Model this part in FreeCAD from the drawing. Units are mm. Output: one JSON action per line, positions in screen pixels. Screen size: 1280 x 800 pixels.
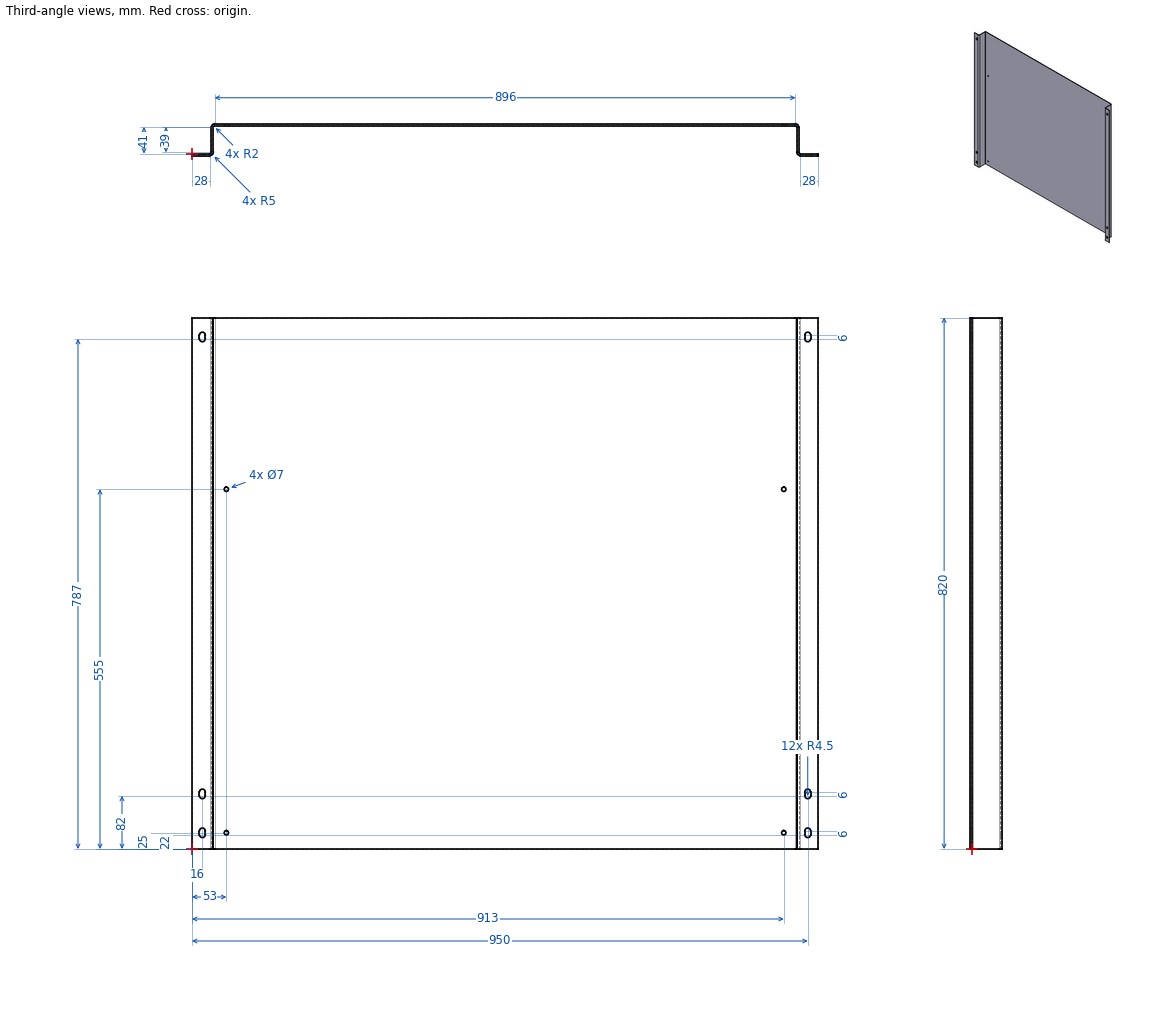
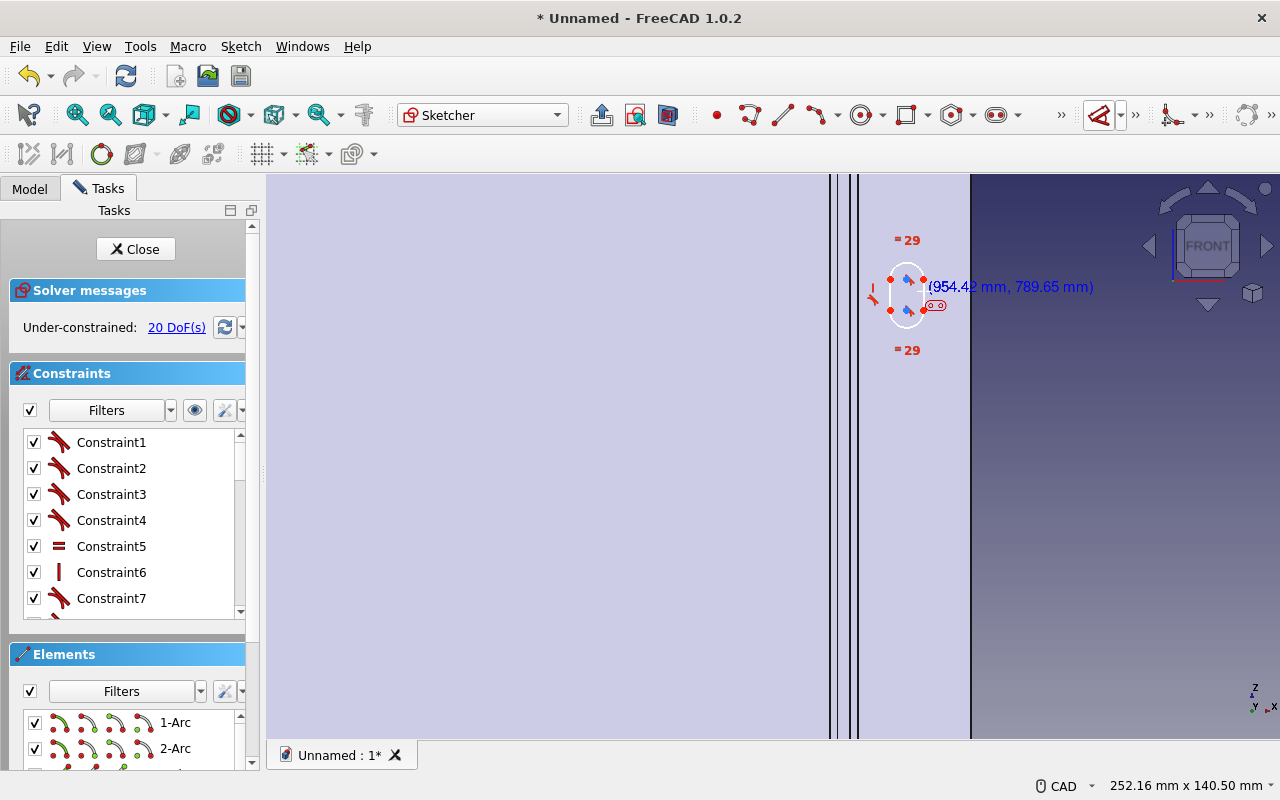
{"action": "scroll", "coordinate": [916, 281], "scroll_direction": "down", "scroll_amount": 11}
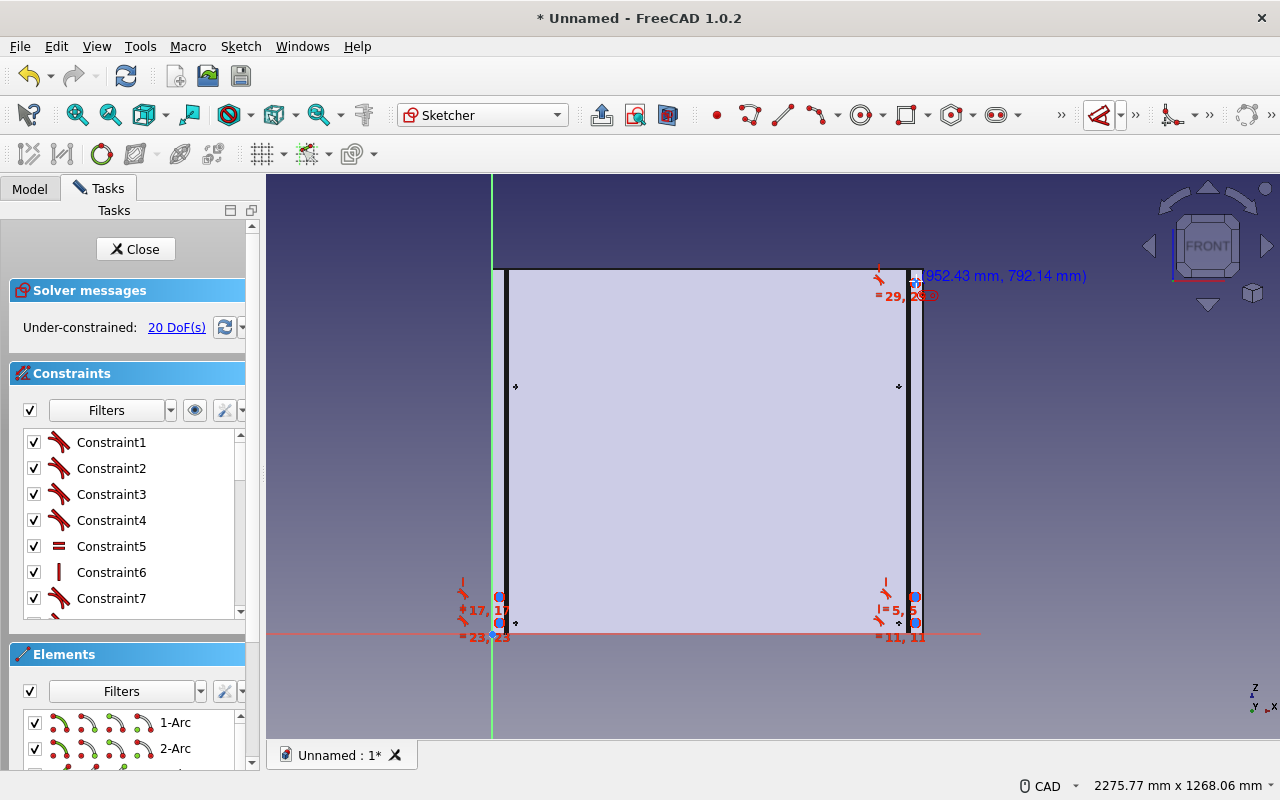
{"action": "scroll", "coordinate": [499, 284], "scroll_direction": "up", "scroll_amount": 13}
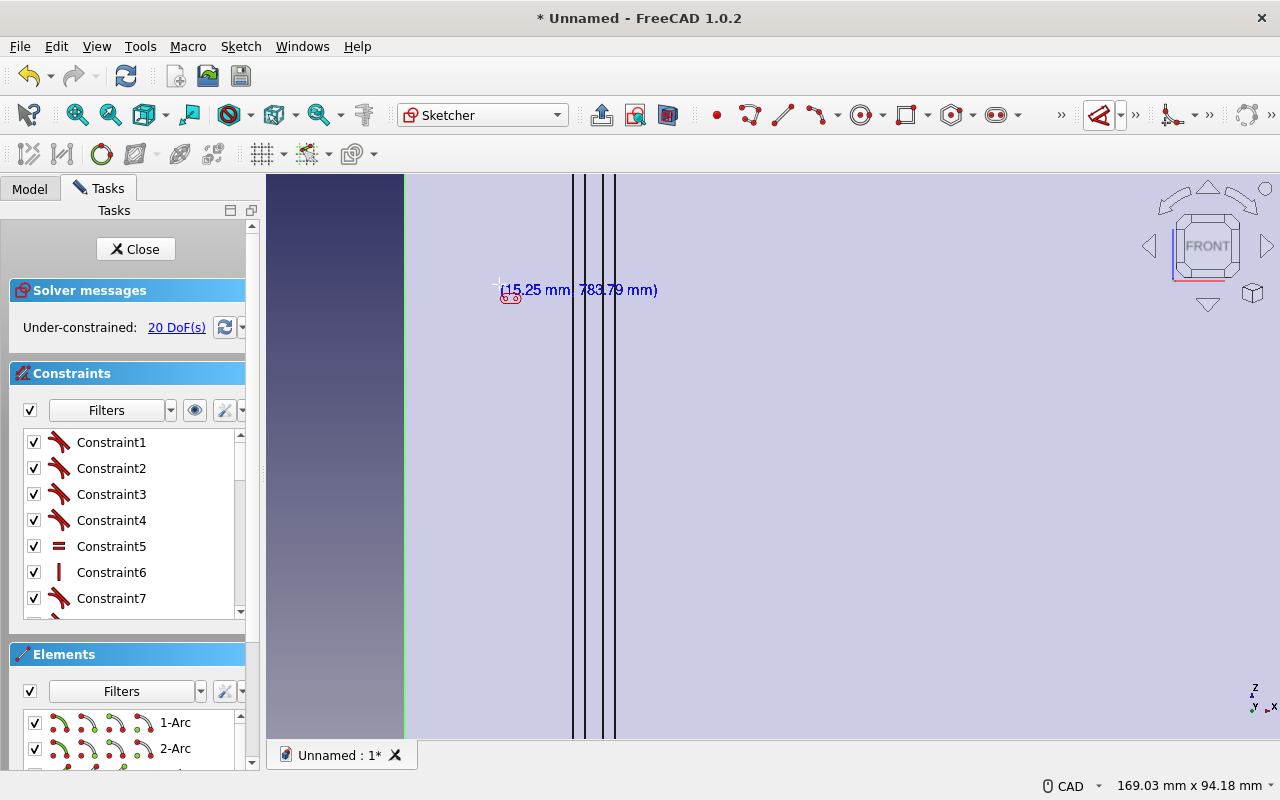
{"action": "scroll", "coordinate": [499, 284], "scroll_direction": "down", "scroll_amount": 13}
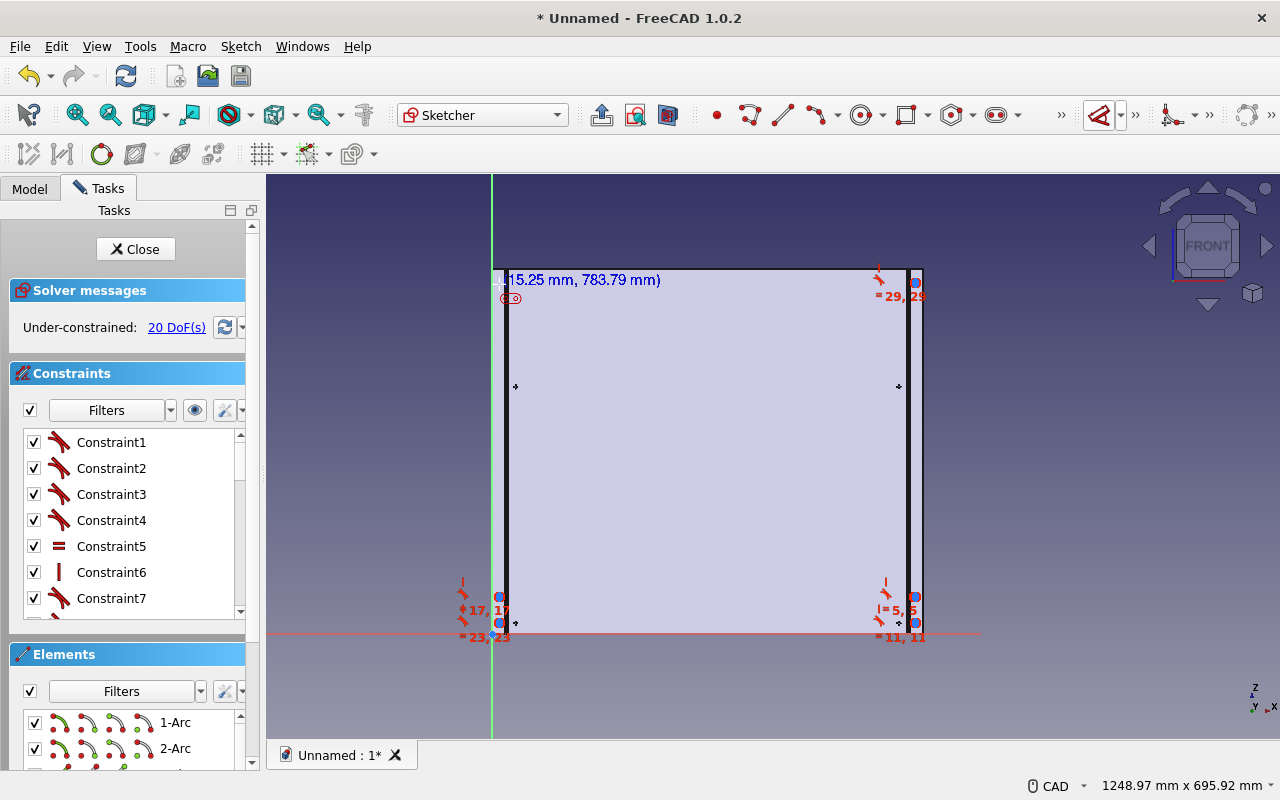
{"action": "scroll", "coordinate": [499, 284], "scroll_direction": "up", "scroll_amount": 5}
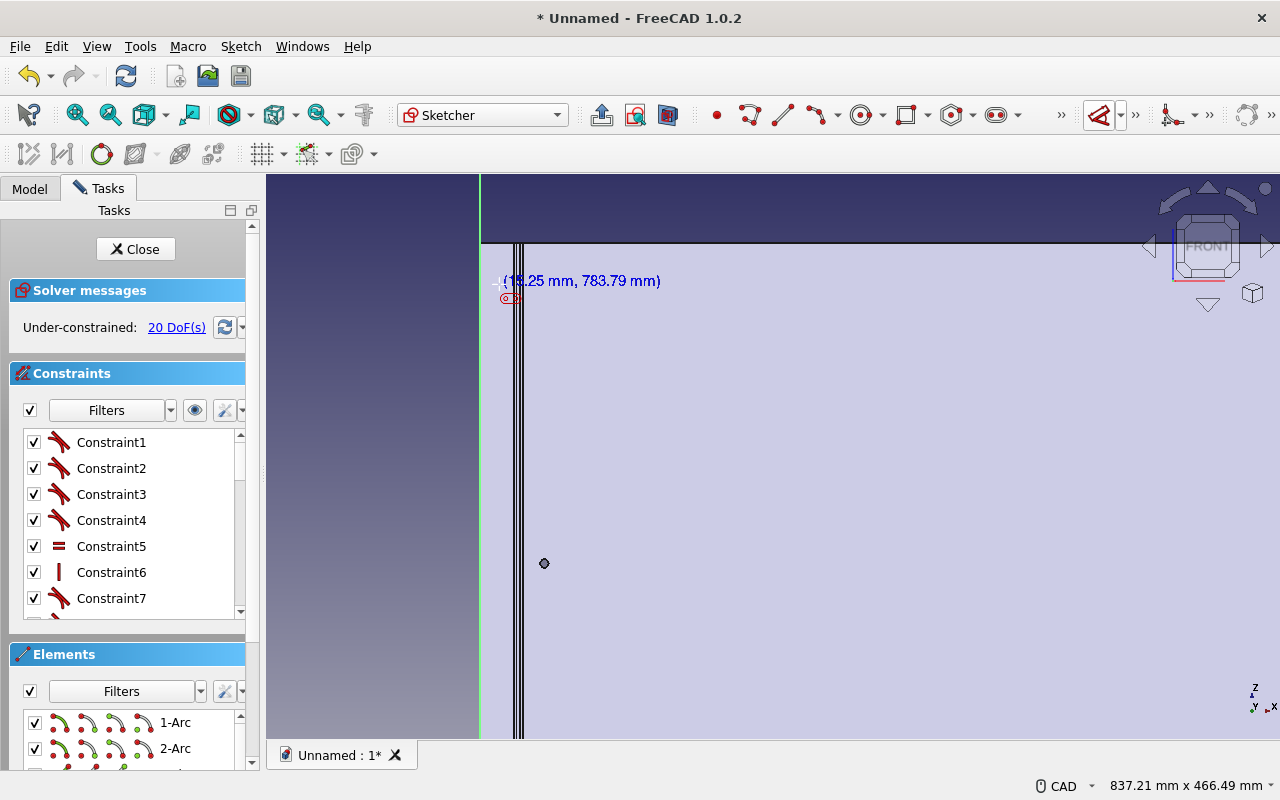
{"action": "left_click", "coordinate": [500, 282]}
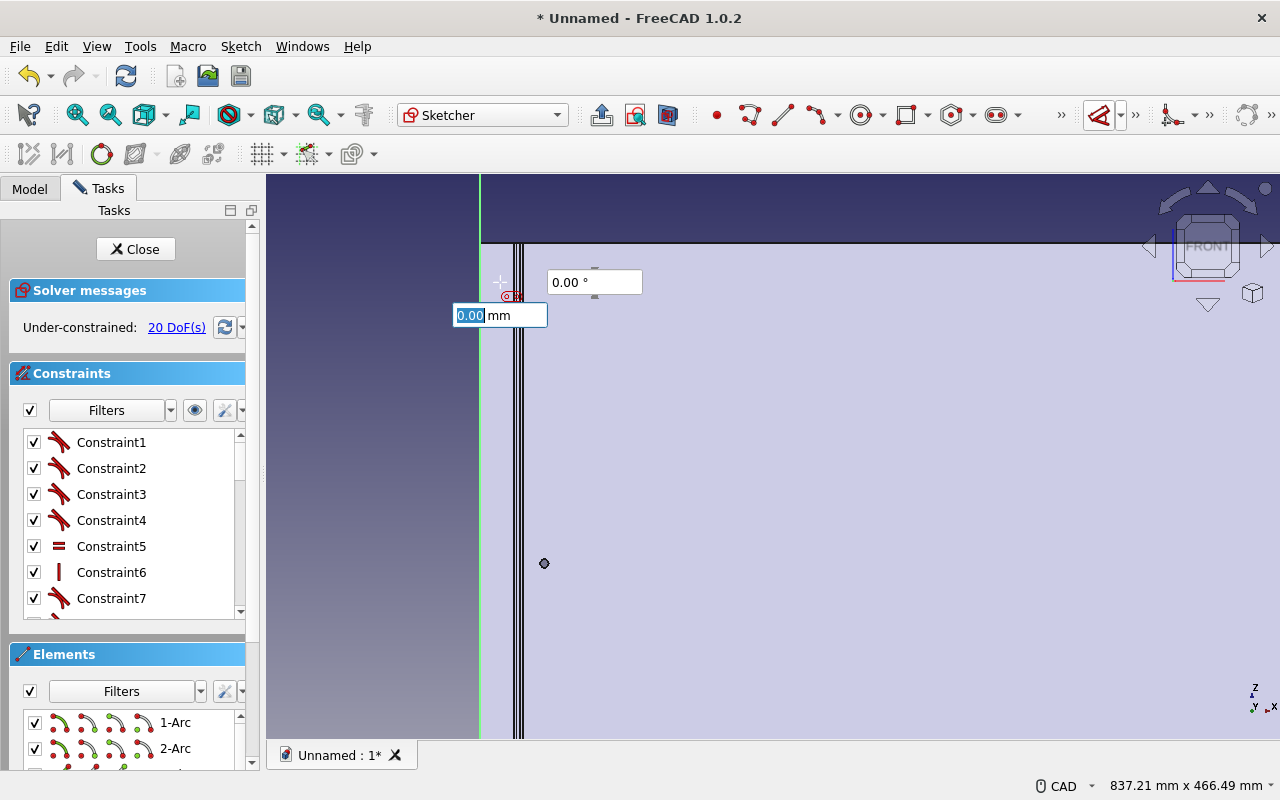
{"action": "scroll", "coordinate": [500, 275], "scroll_direction": "up", "scroll_amount": 4}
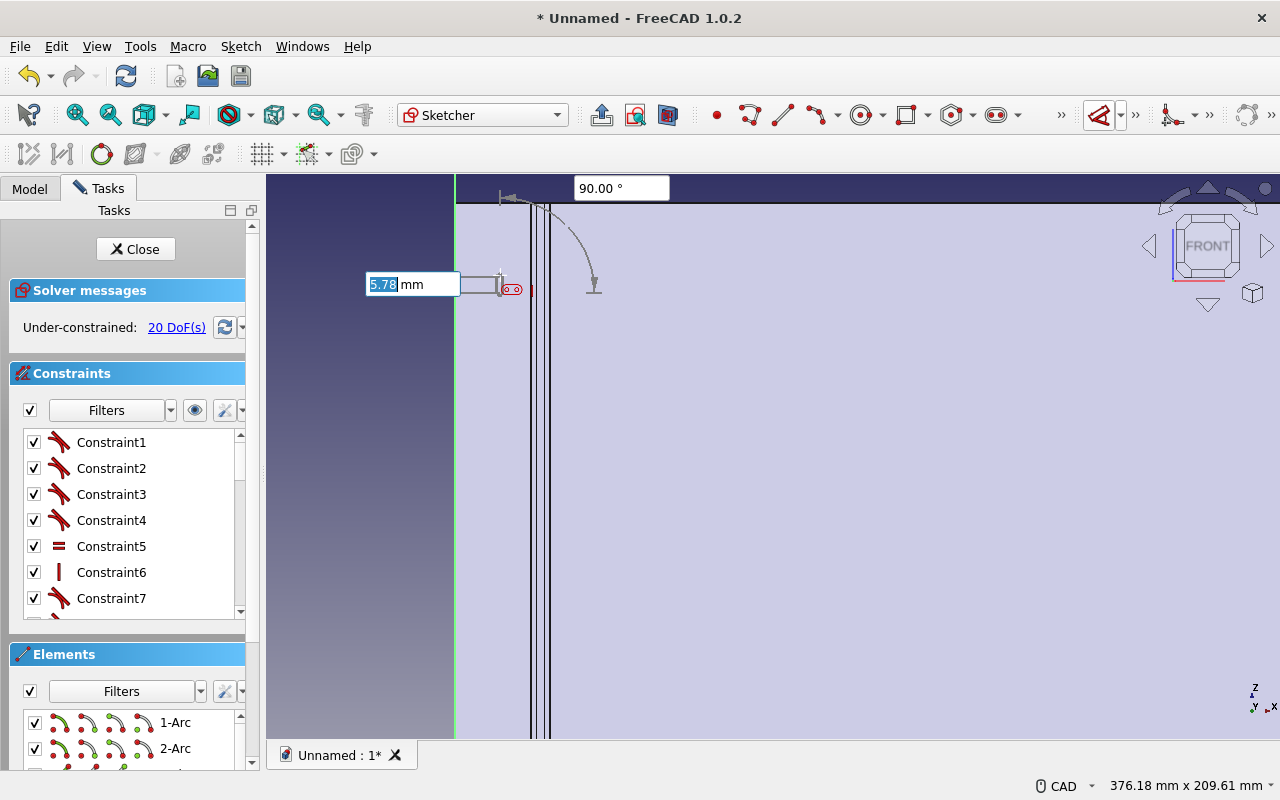
{"action": "left_click", "coordinate": [500, 275]}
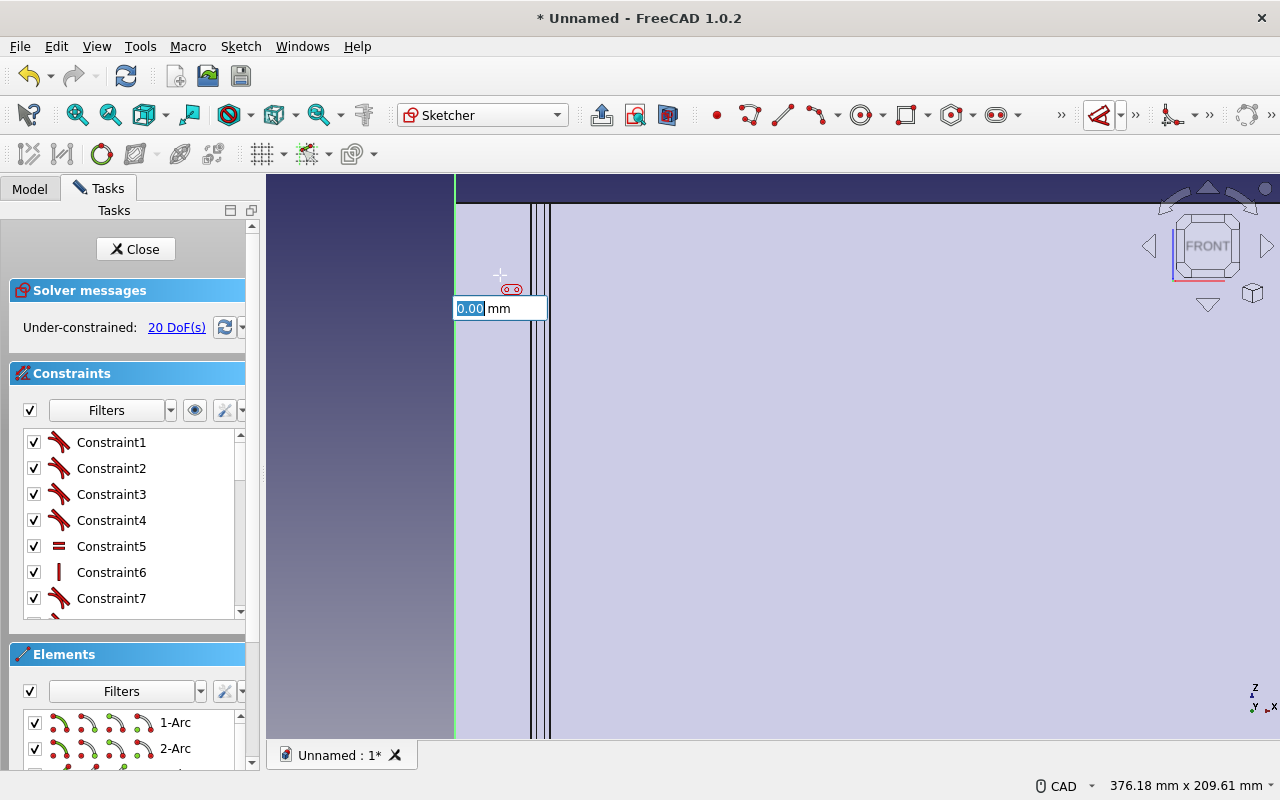
{"action": "scroll", "coordinate": [486, 283], "scroll_direction": "up", "scroll_amount": 2}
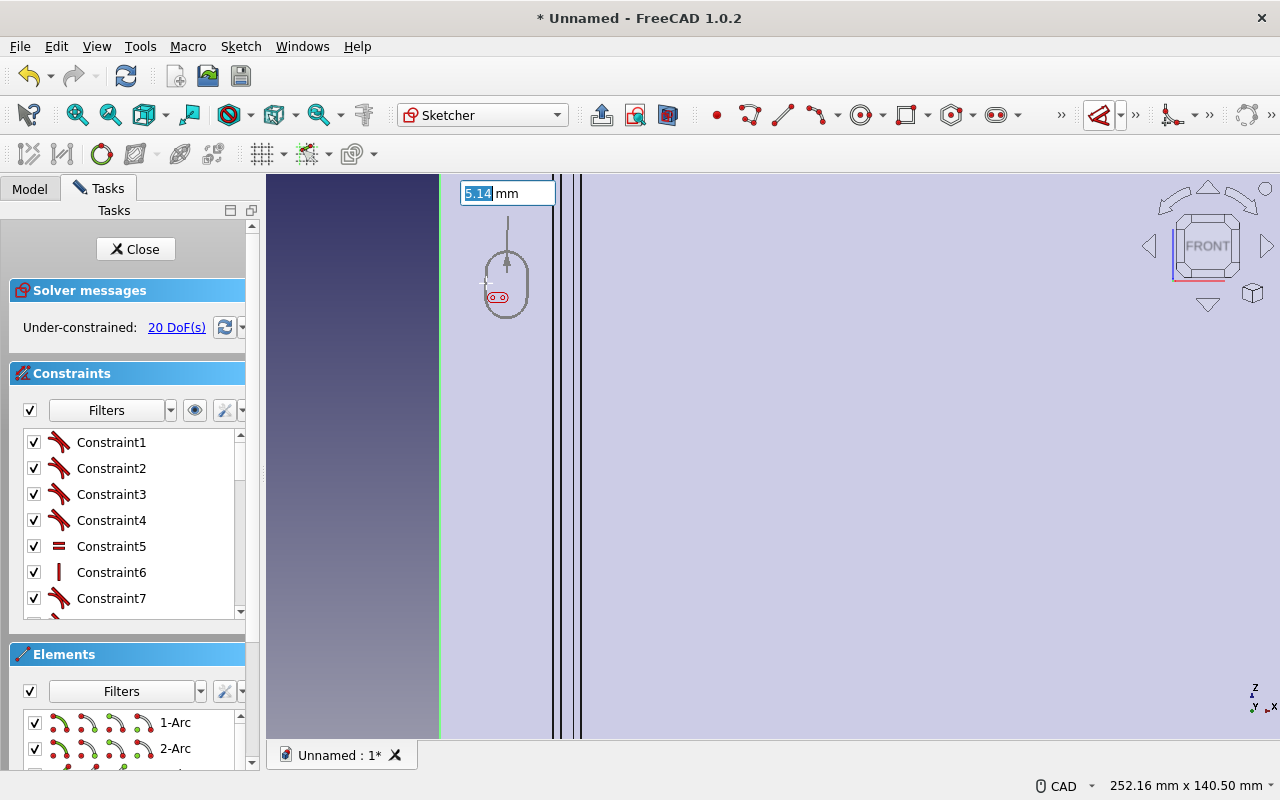
{"action": "left_click", "coordinate": [487, 283]}
{"action": "key", "text": "Escape"}